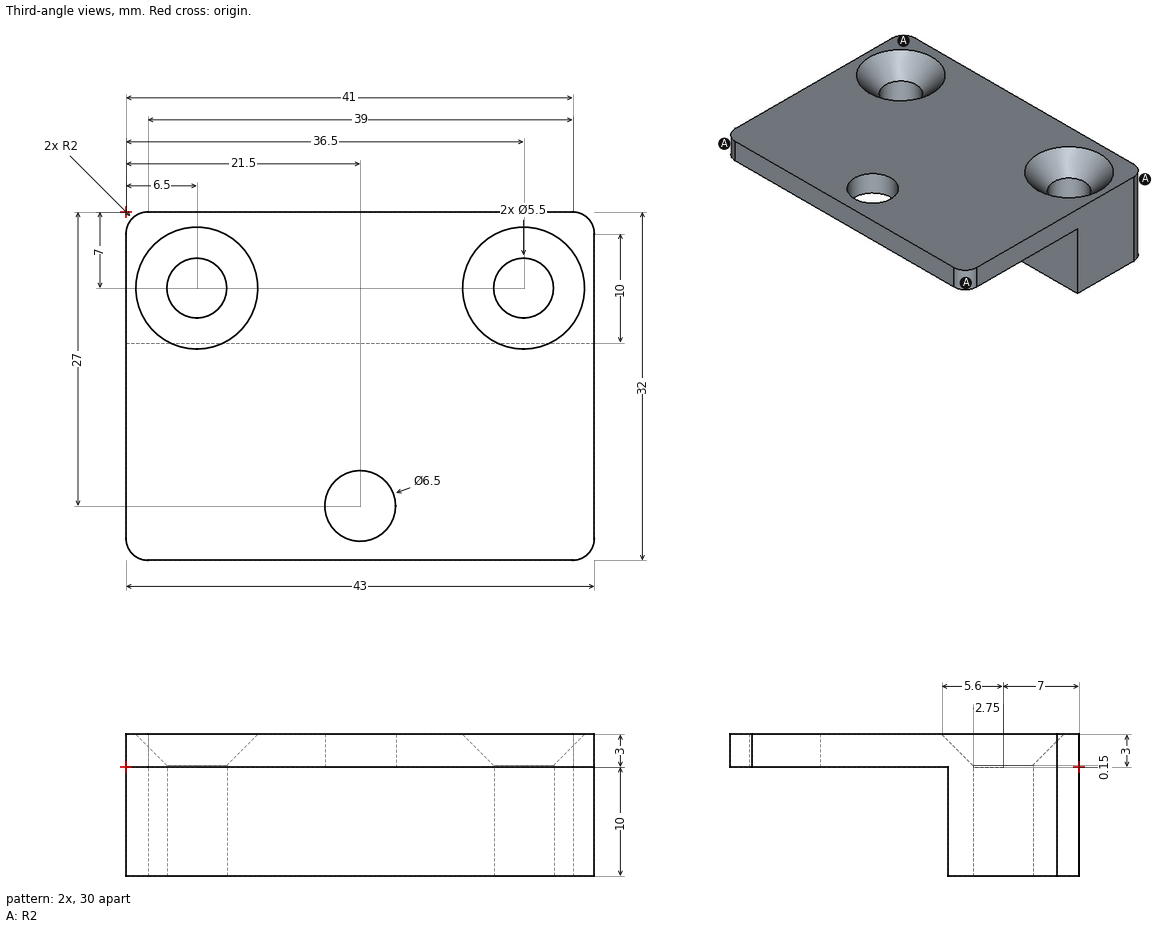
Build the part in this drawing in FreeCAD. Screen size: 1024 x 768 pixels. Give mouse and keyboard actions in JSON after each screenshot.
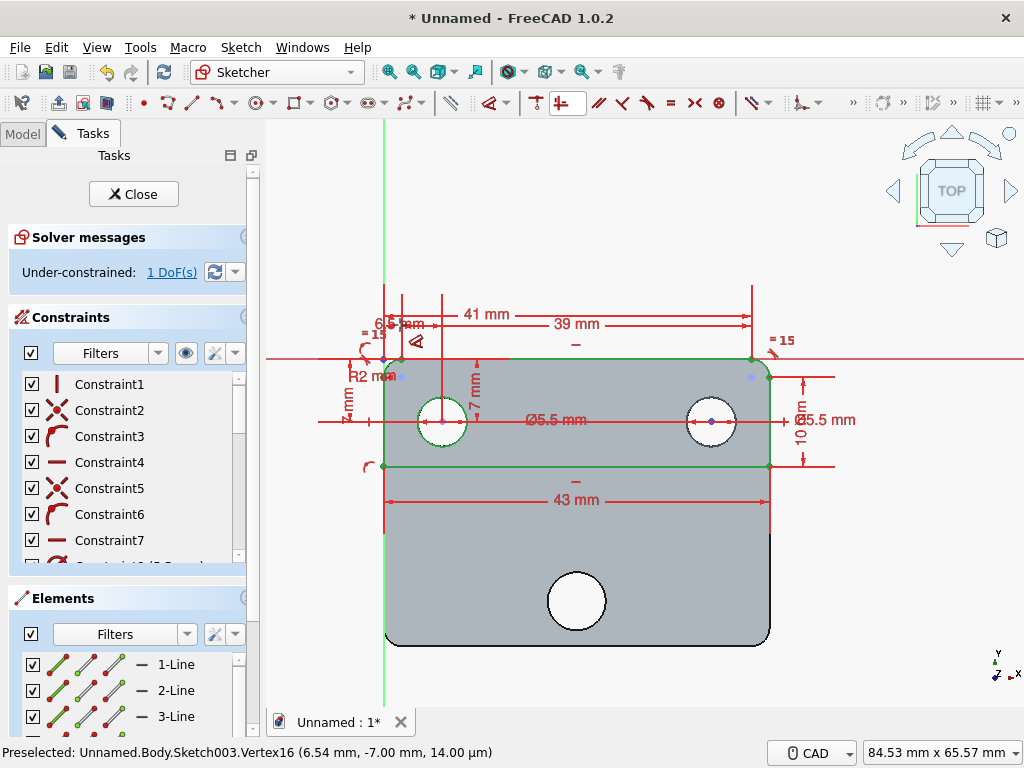
{"action": "left_click", "coordinate": [711, 422]}
{"action": "left_click", "coordinate": [662, 325]}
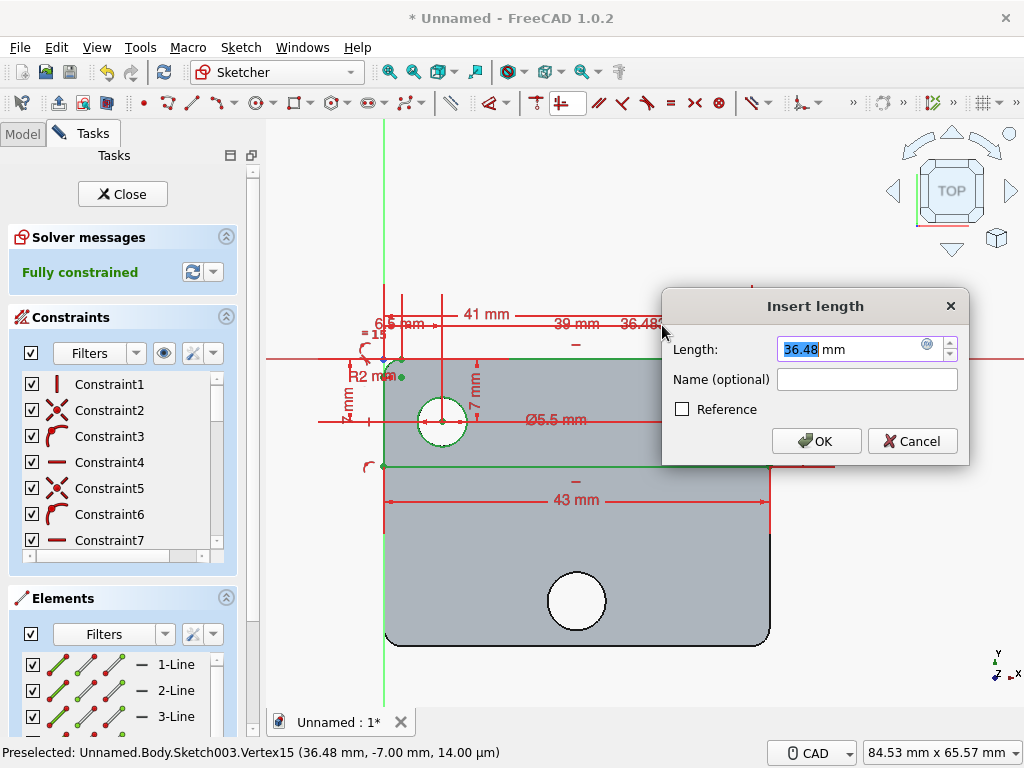
{"action": "type", "text": "36.5"}
{"action": "key", "text": "Return"}
{"action": "key", "text": "Escape"}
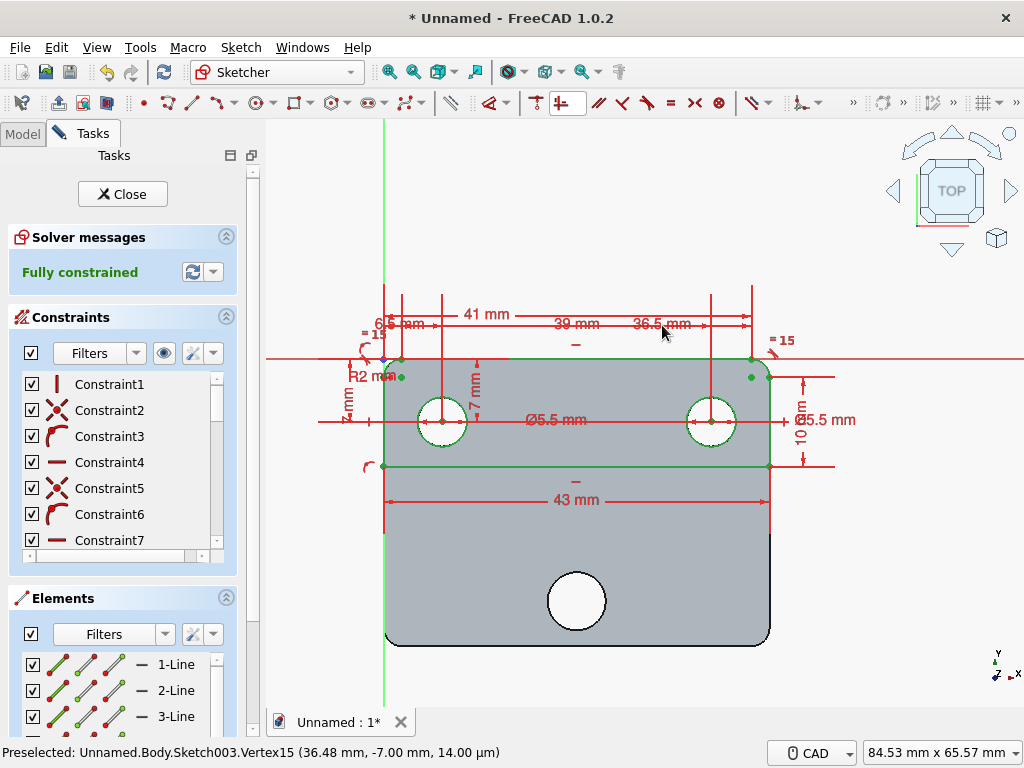
{"action": "left_click", "coordinate": [123, 194]}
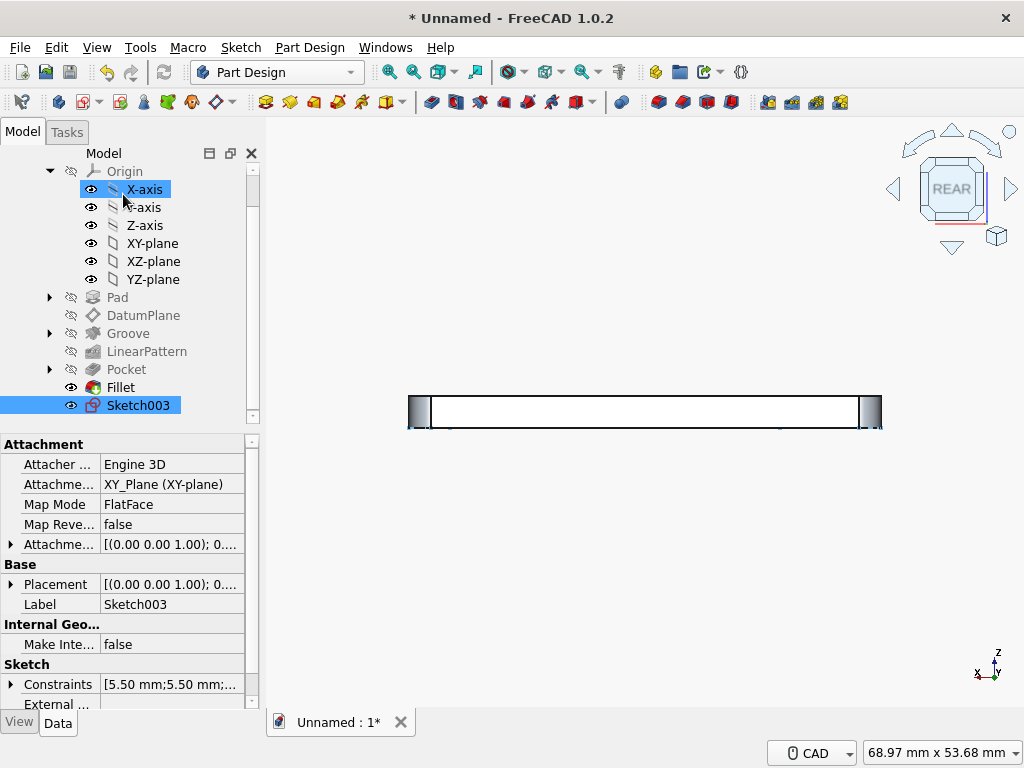
{"action": "left_click", "coordinate": [266, 102]}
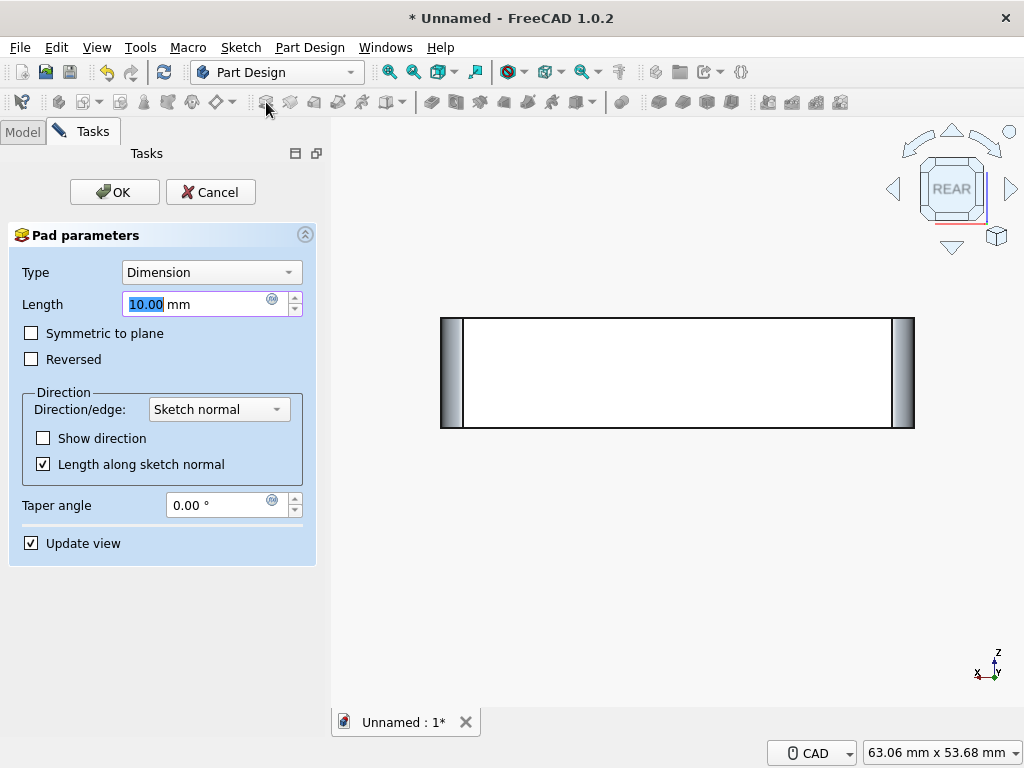
{"action": "type", "text": "10"}
{"action": "key", "text": "Tab"}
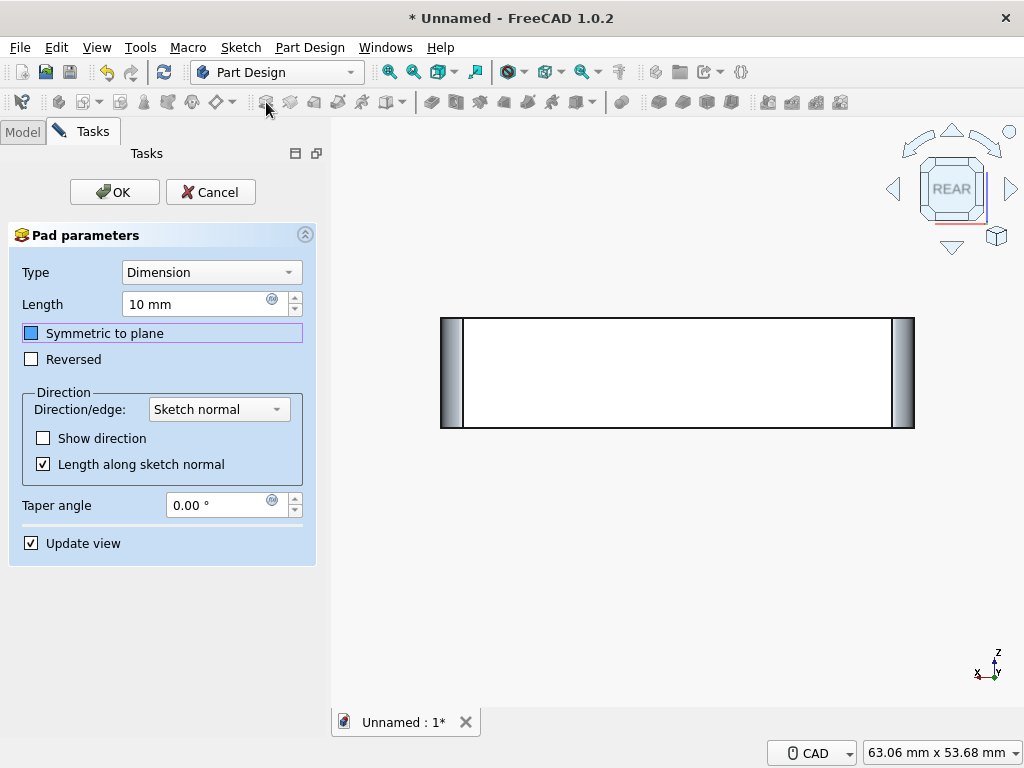
{"action": "left_click", "coordinate": [30, 359]}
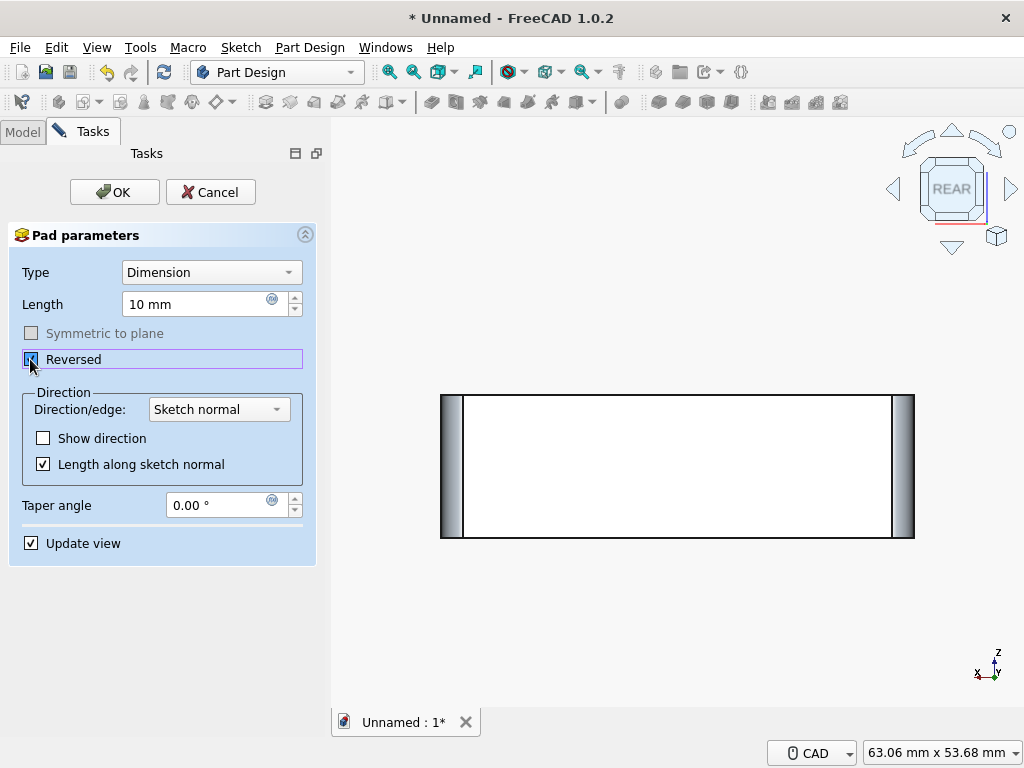
{"action": "left_click", "coordinate": [115, 192]}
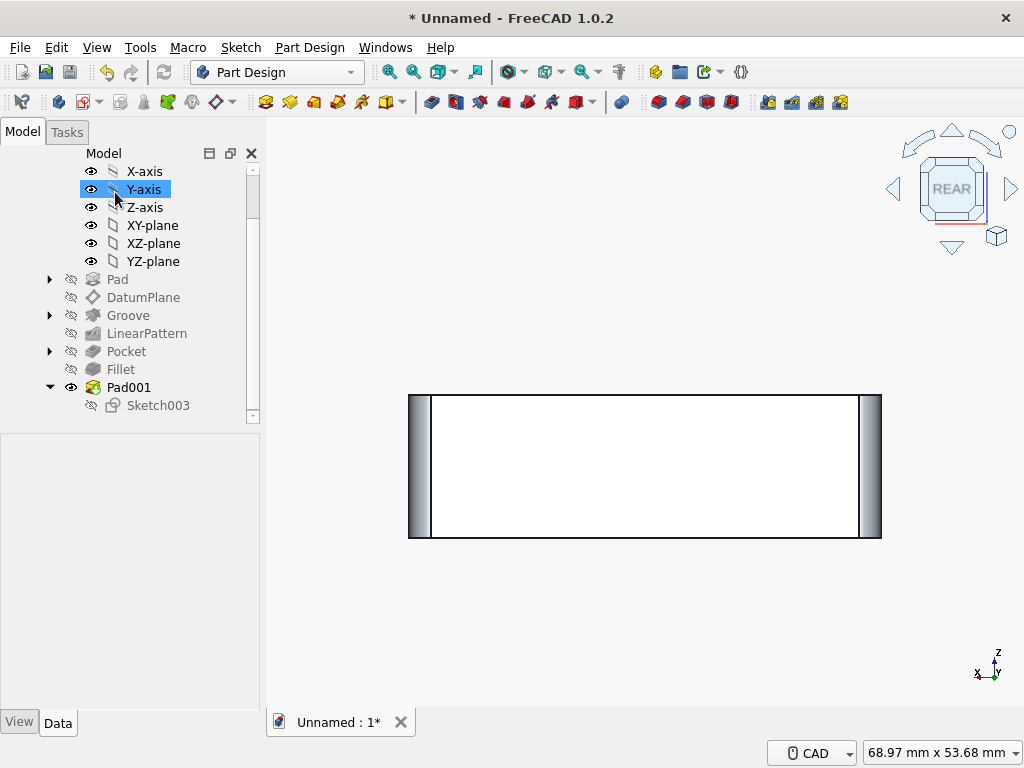
{"action": "key", "text": "0"}